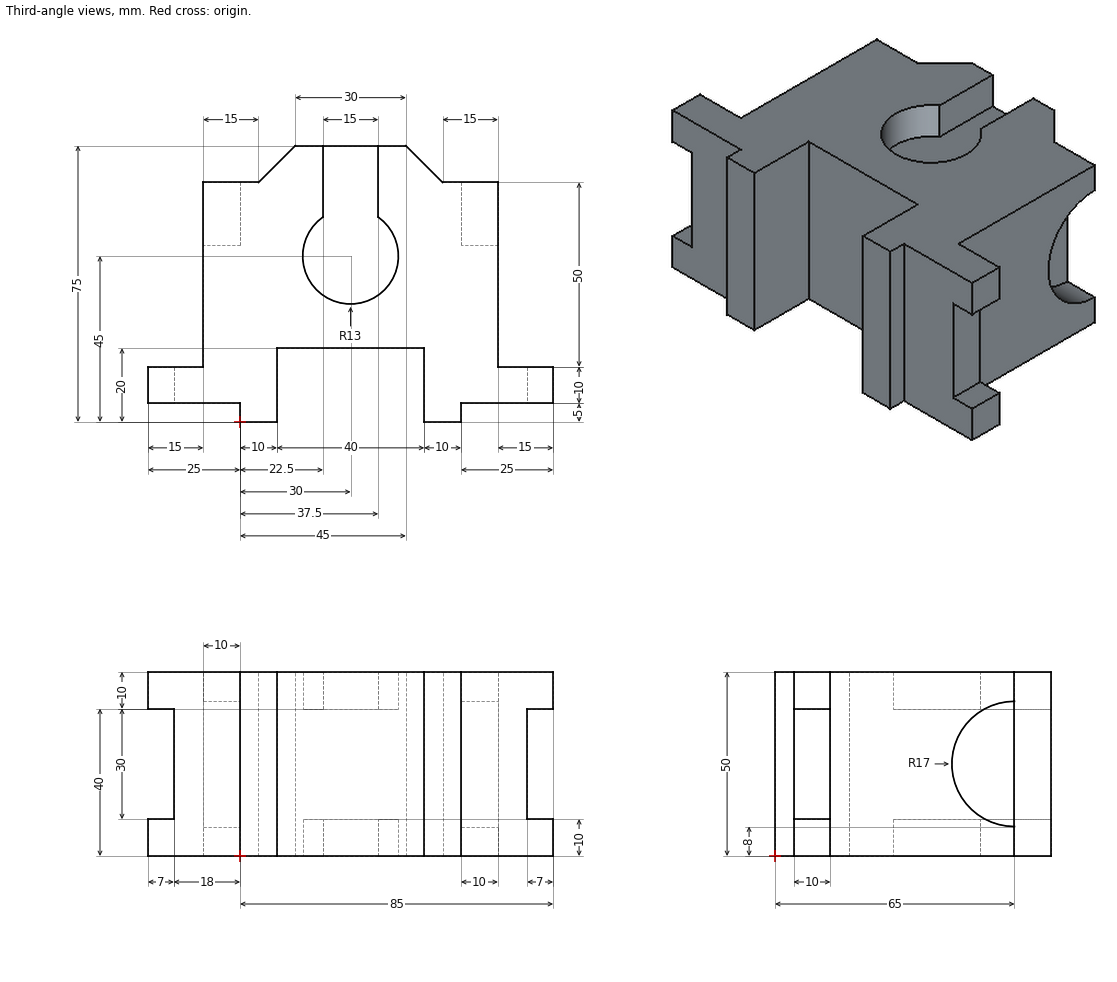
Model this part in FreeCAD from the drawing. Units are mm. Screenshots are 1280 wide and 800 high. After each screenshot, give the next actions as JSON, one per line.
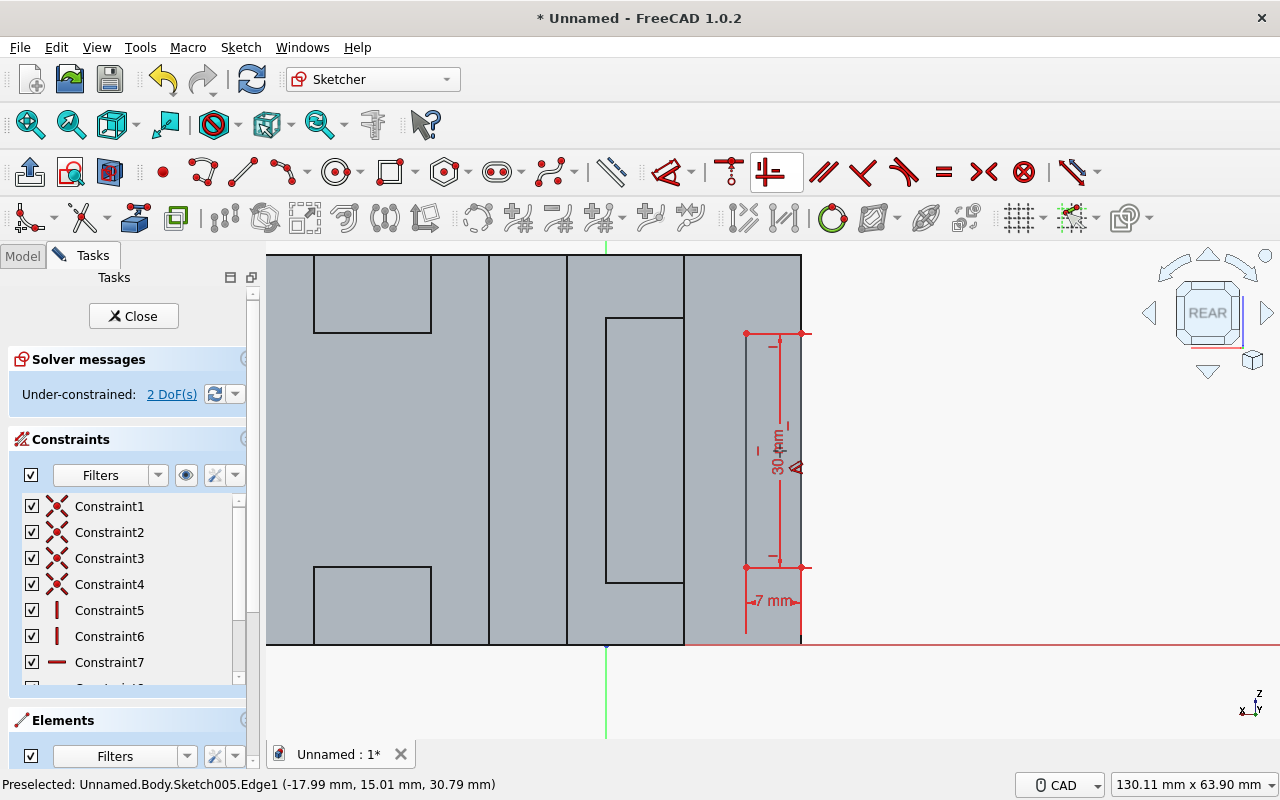
{"action": "left_click", "coordinate": [746, 334]}
{"action": "left_click", "coordinate": [676, 679]}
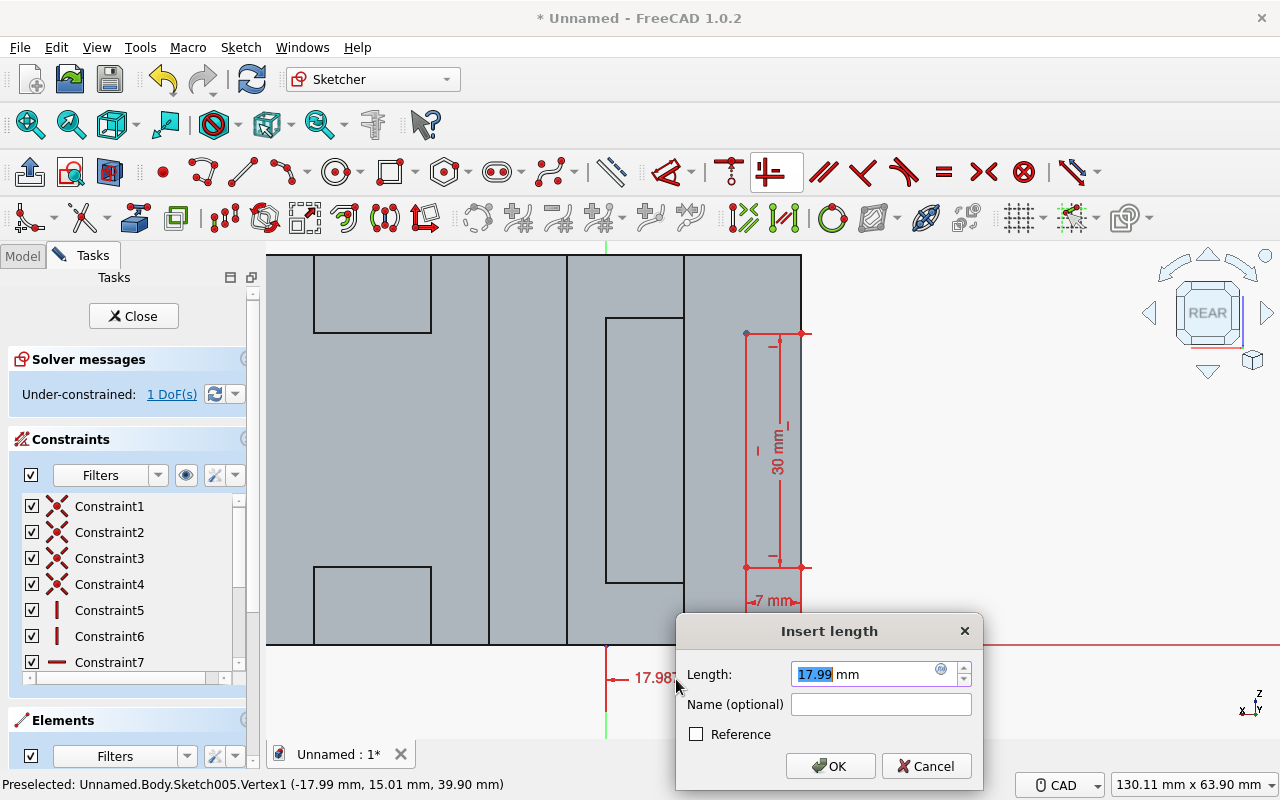
{"action": "type", "text": "18"}
{"action": "key", "text": "Return"}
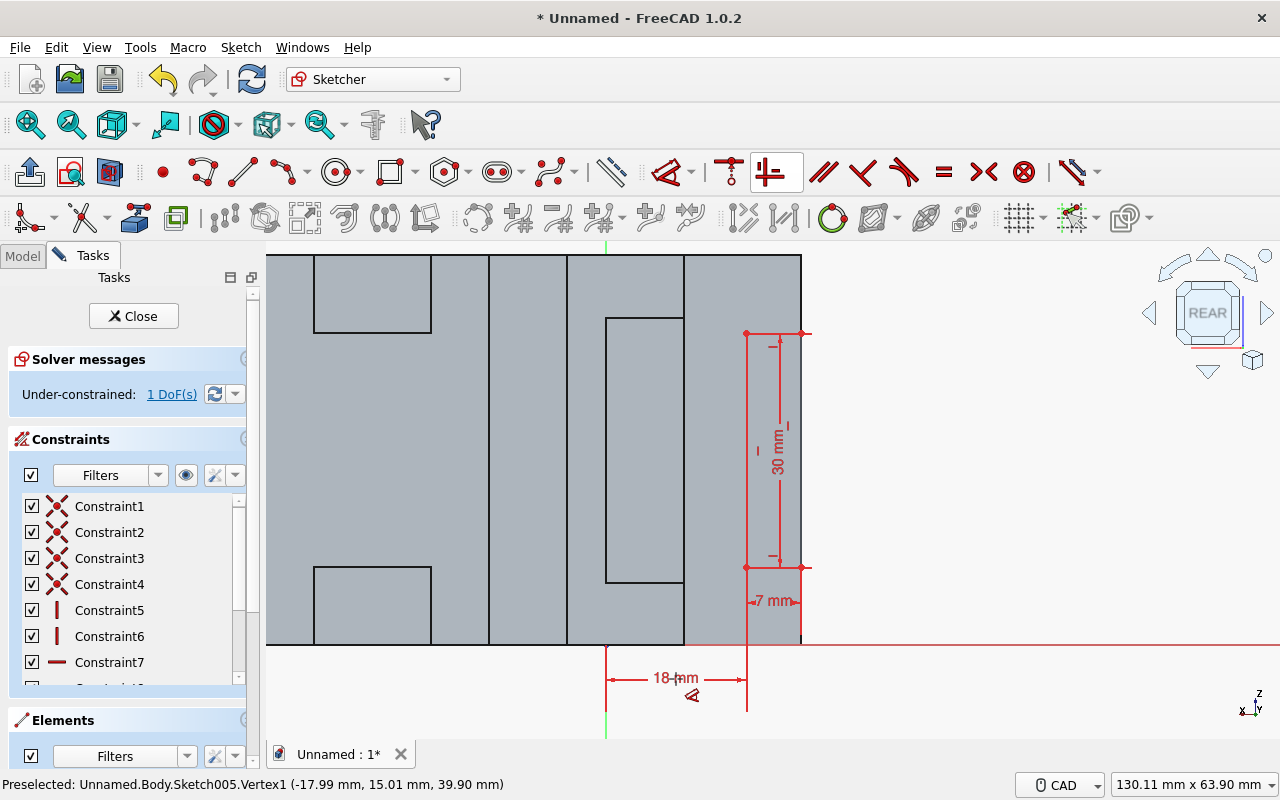
{"action": "left_click", "coordinate": [747, 334]}
{"action": "left_click", "coordinate": [572, 489]}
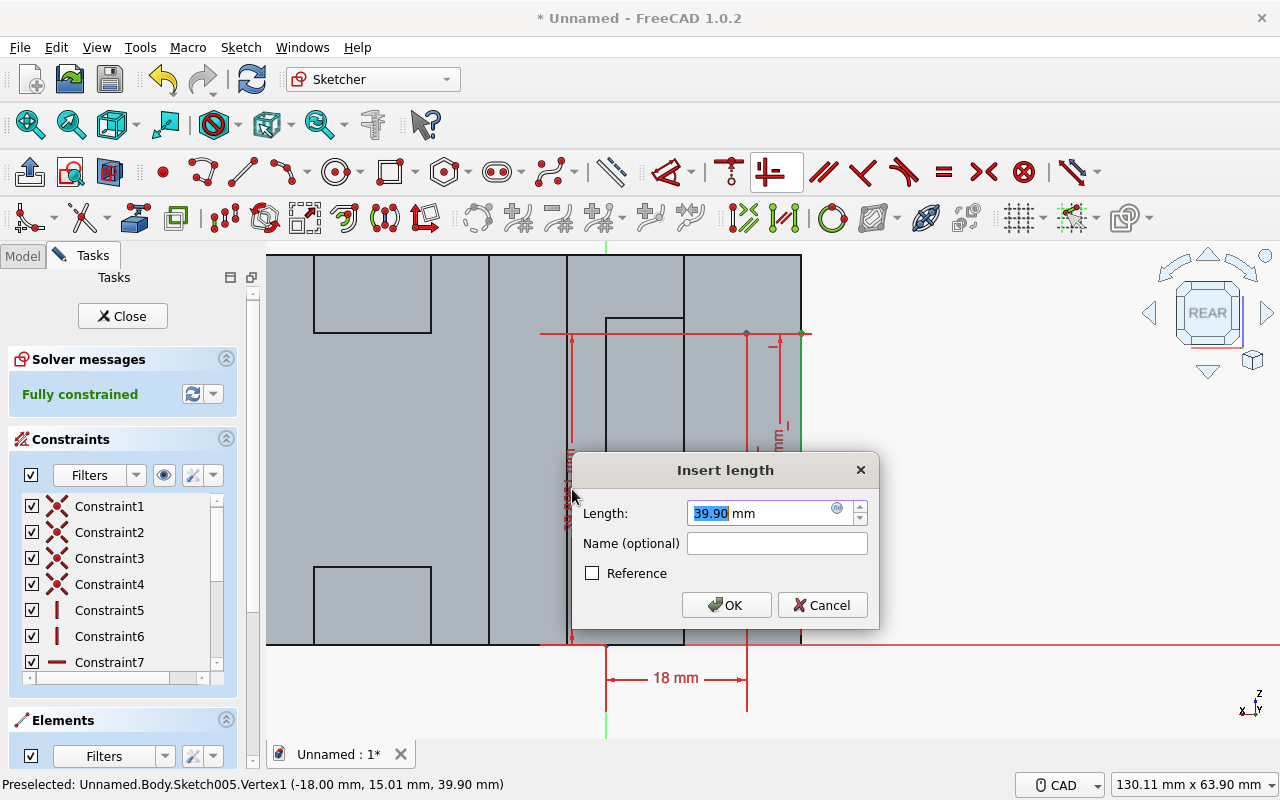
{"action": "type", "text": "40"}
{"action": "key", "text": "Return"}
{"action": "key", "text": "Escape"}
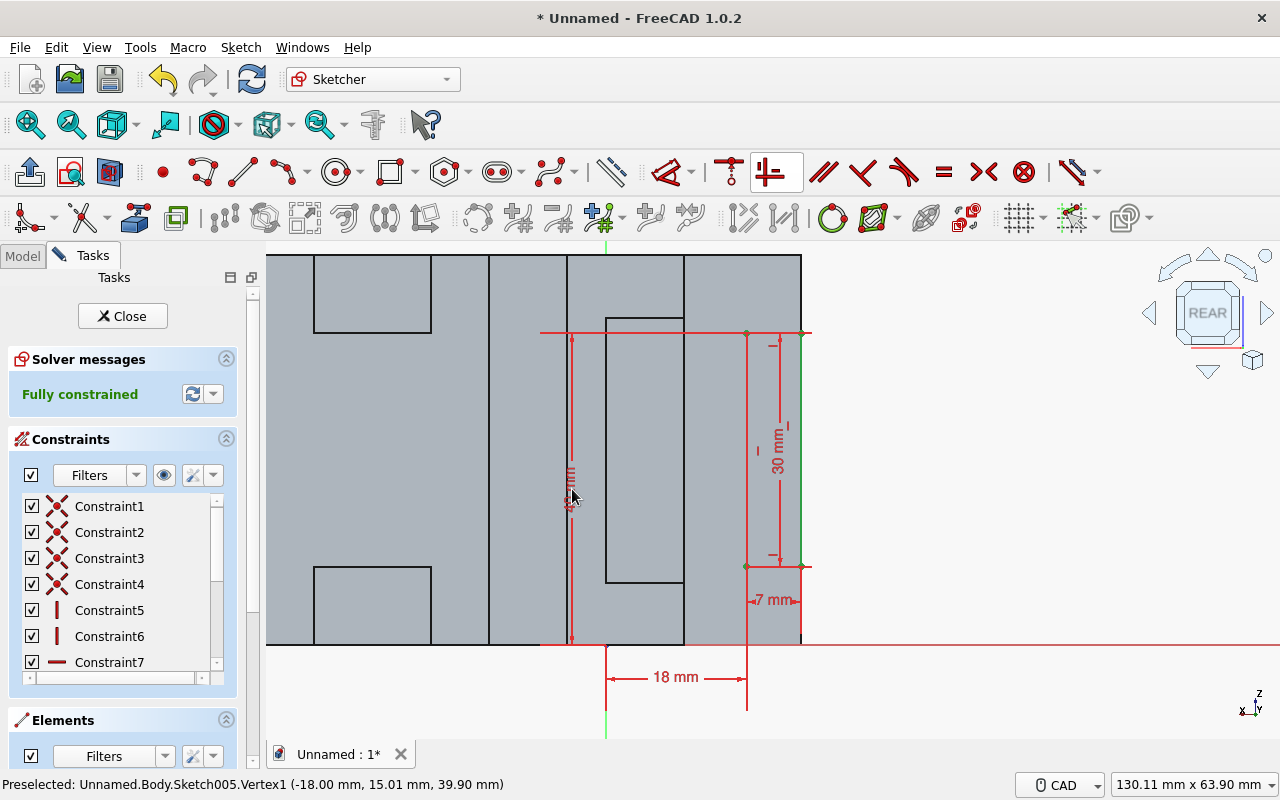
{"action": "left_click", "coordinate": [123, 316]}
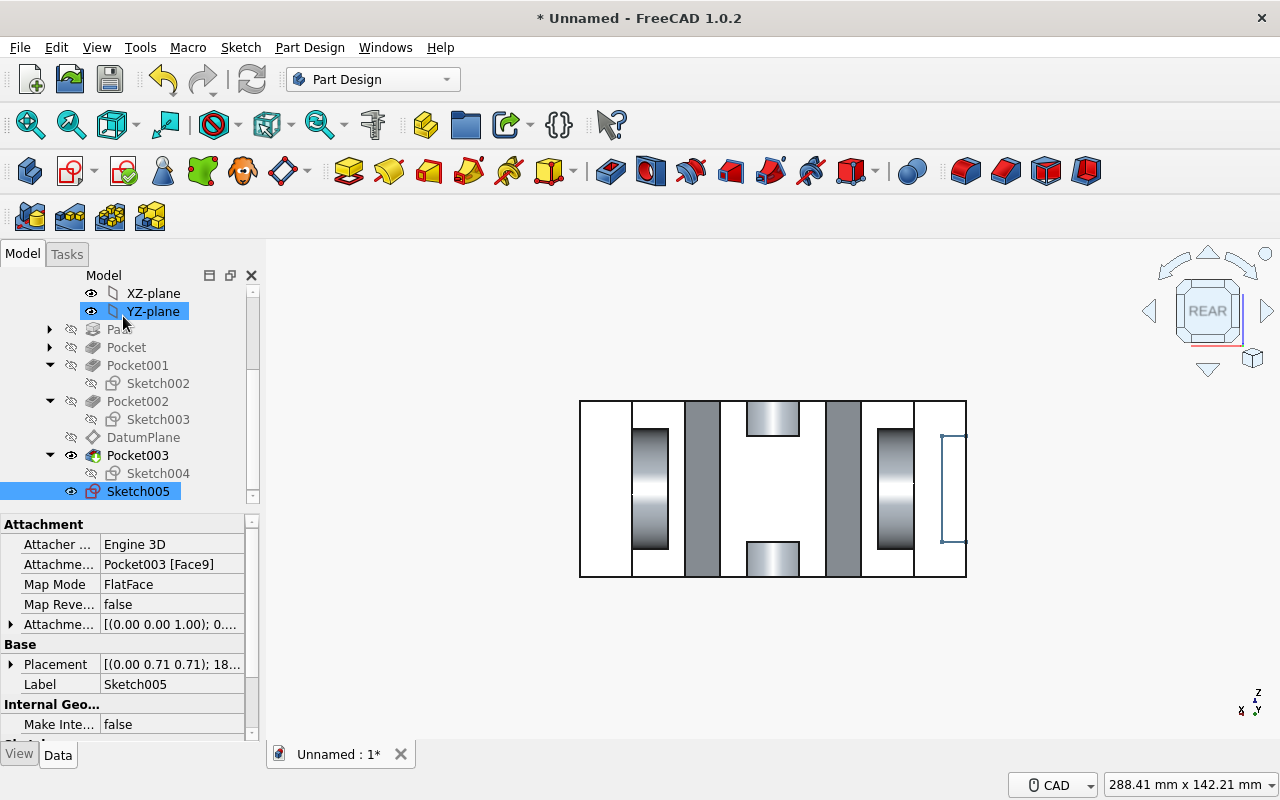
{"action": "left_click", "coordinate": [612, 172]}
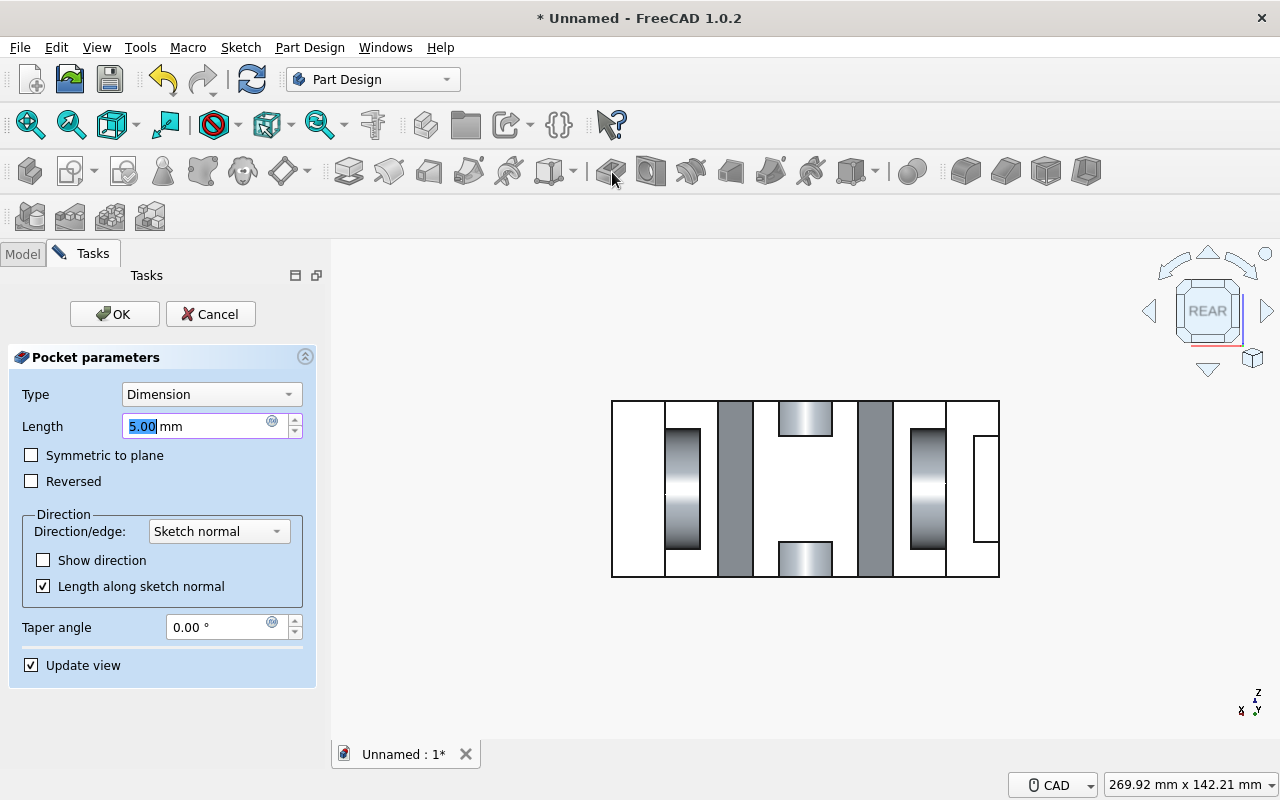
{"action": "type", "text": "10"}
{"action": "key", "text": "Tab"}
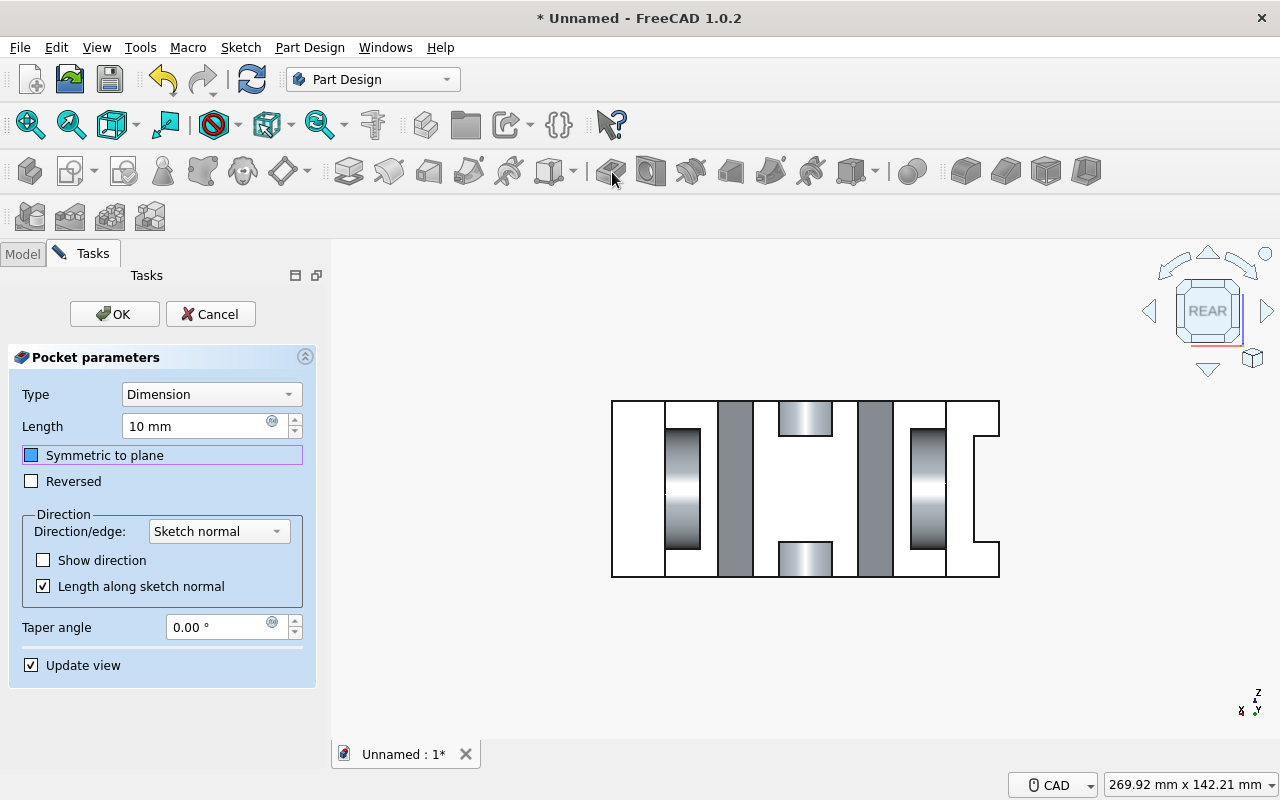
{"action": "left_click", "coordinate": [115, 314]}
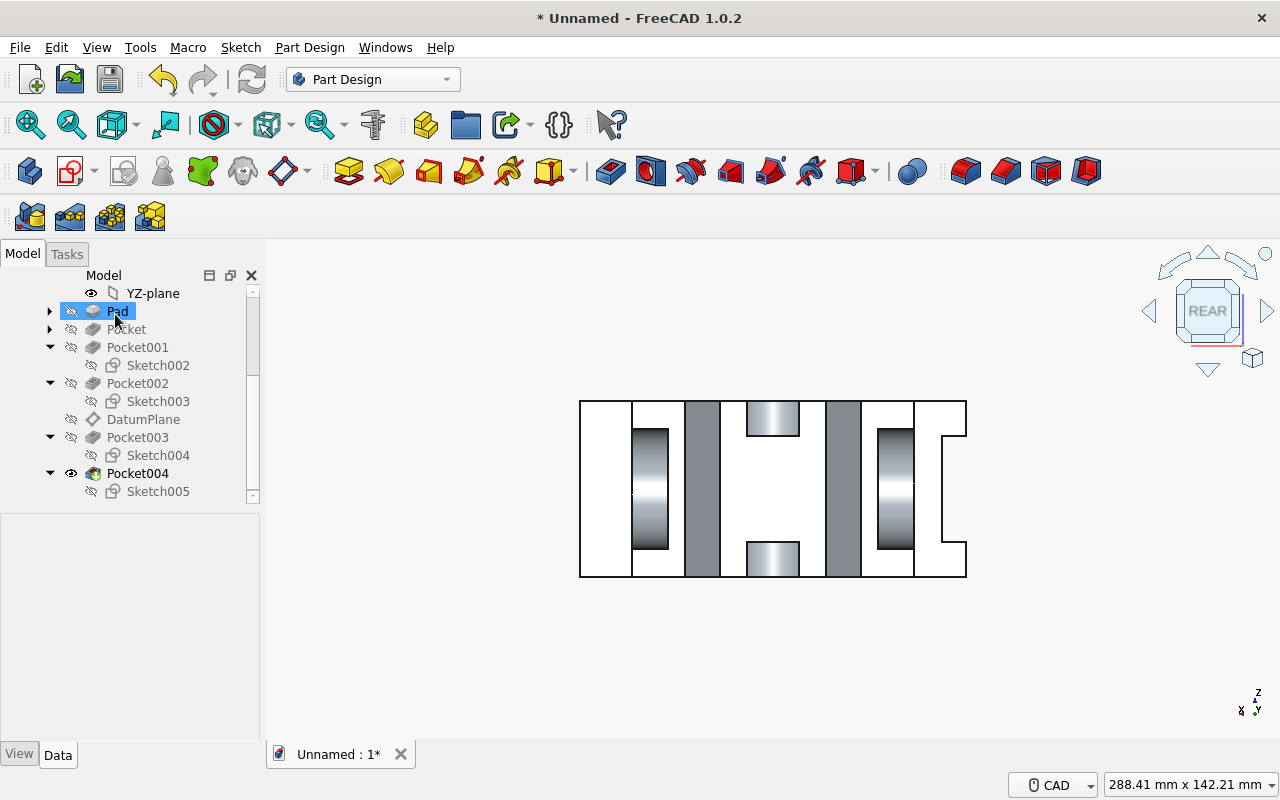
{"action": "left_click", "coordinate": [32, 126]}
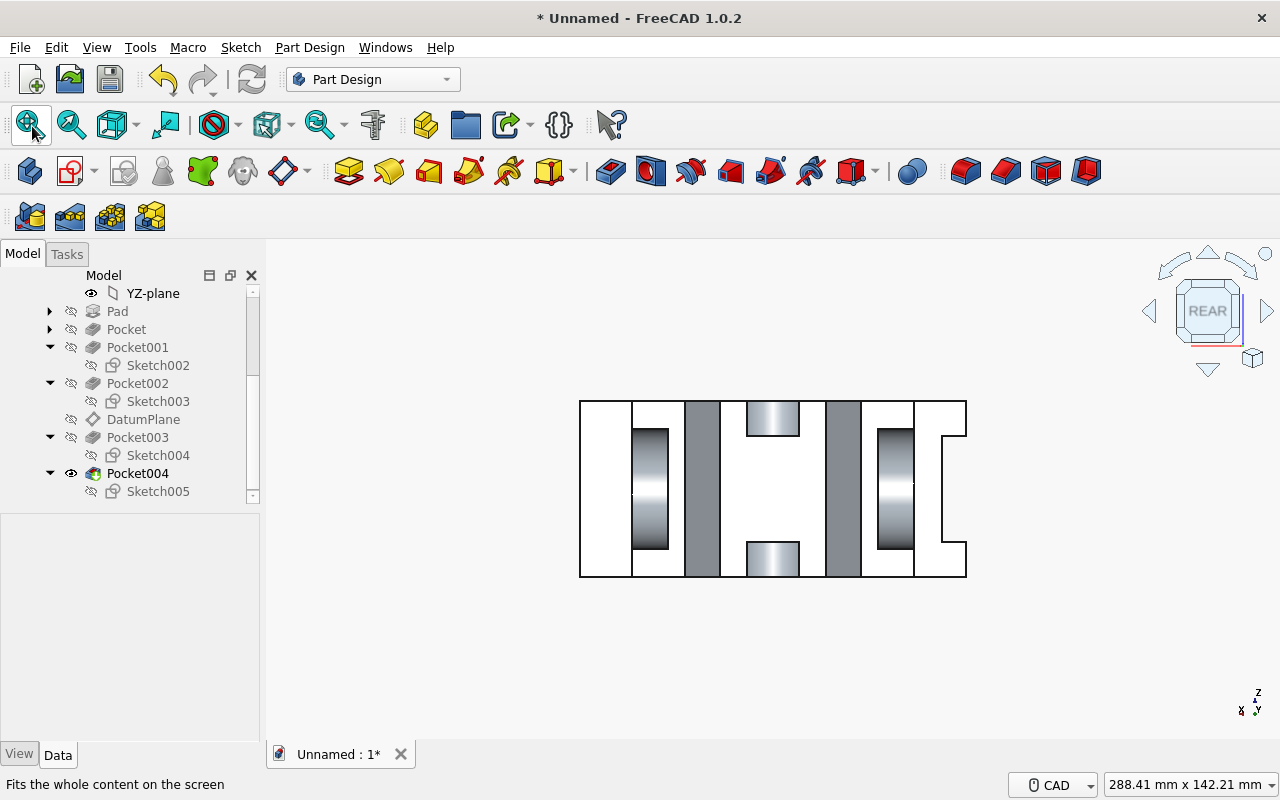
{"action": "left_click", "coordinate": [606, 438]}